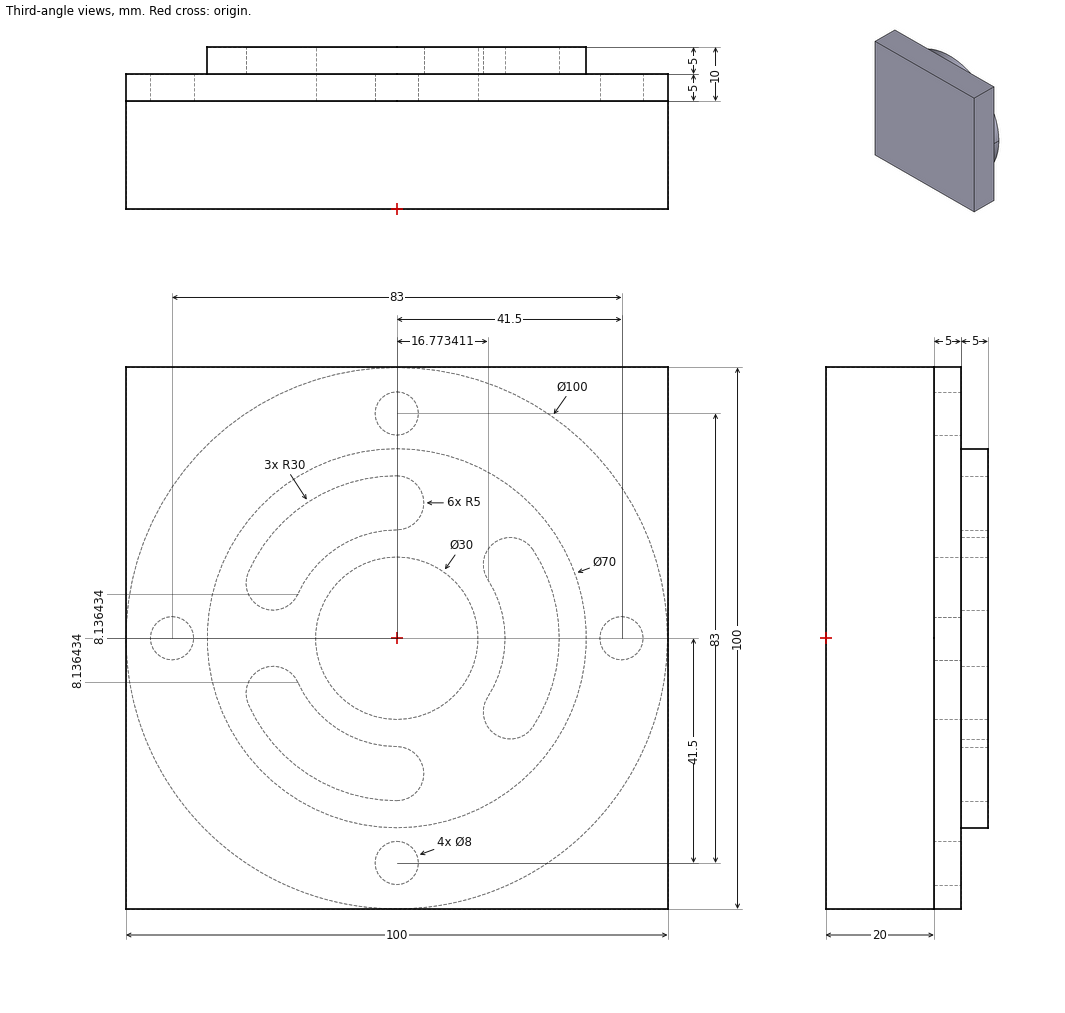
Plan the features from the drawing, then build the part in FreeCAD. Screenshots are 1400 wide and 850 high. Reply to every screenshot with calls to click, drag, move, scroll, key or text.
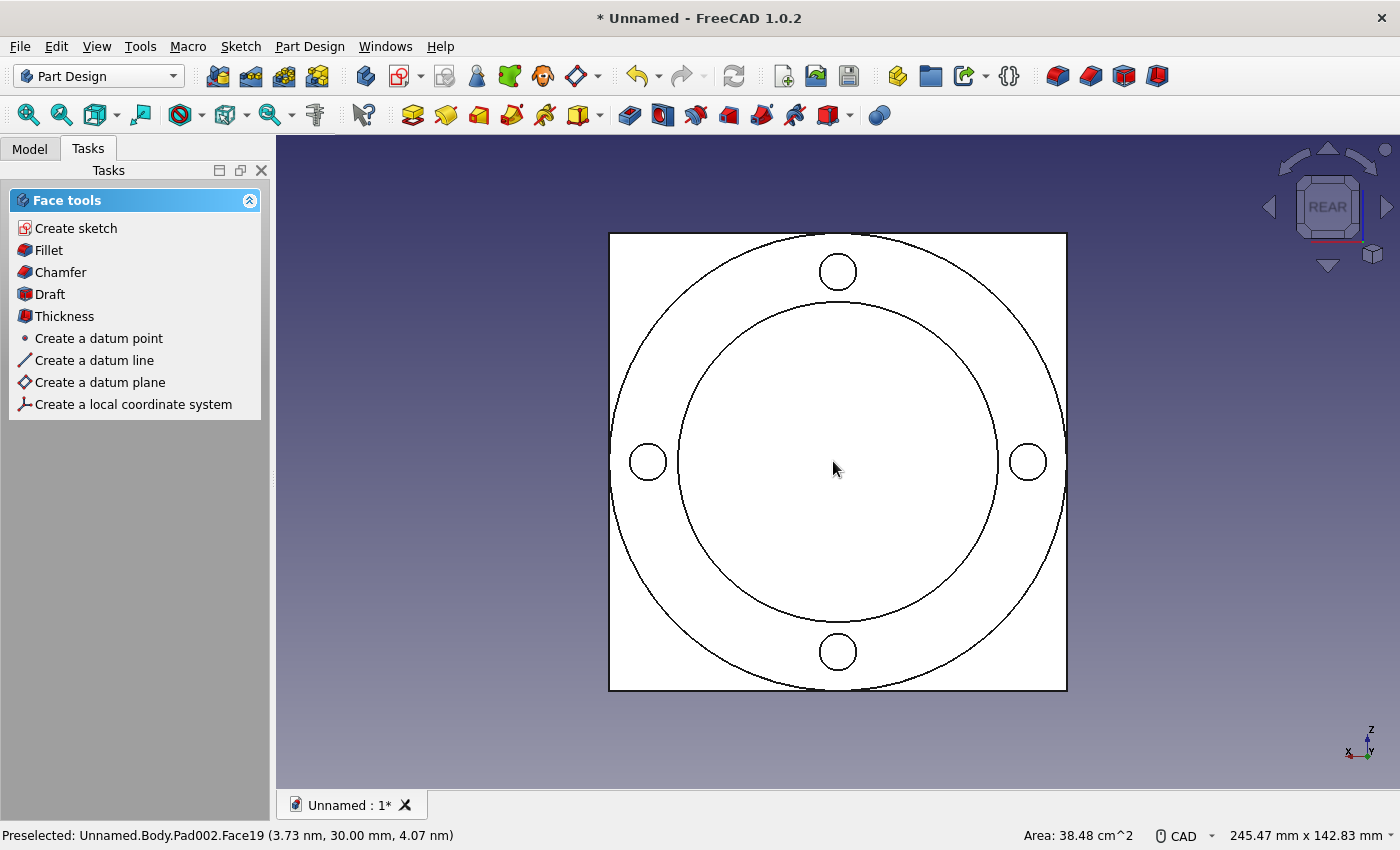
click(398, 76)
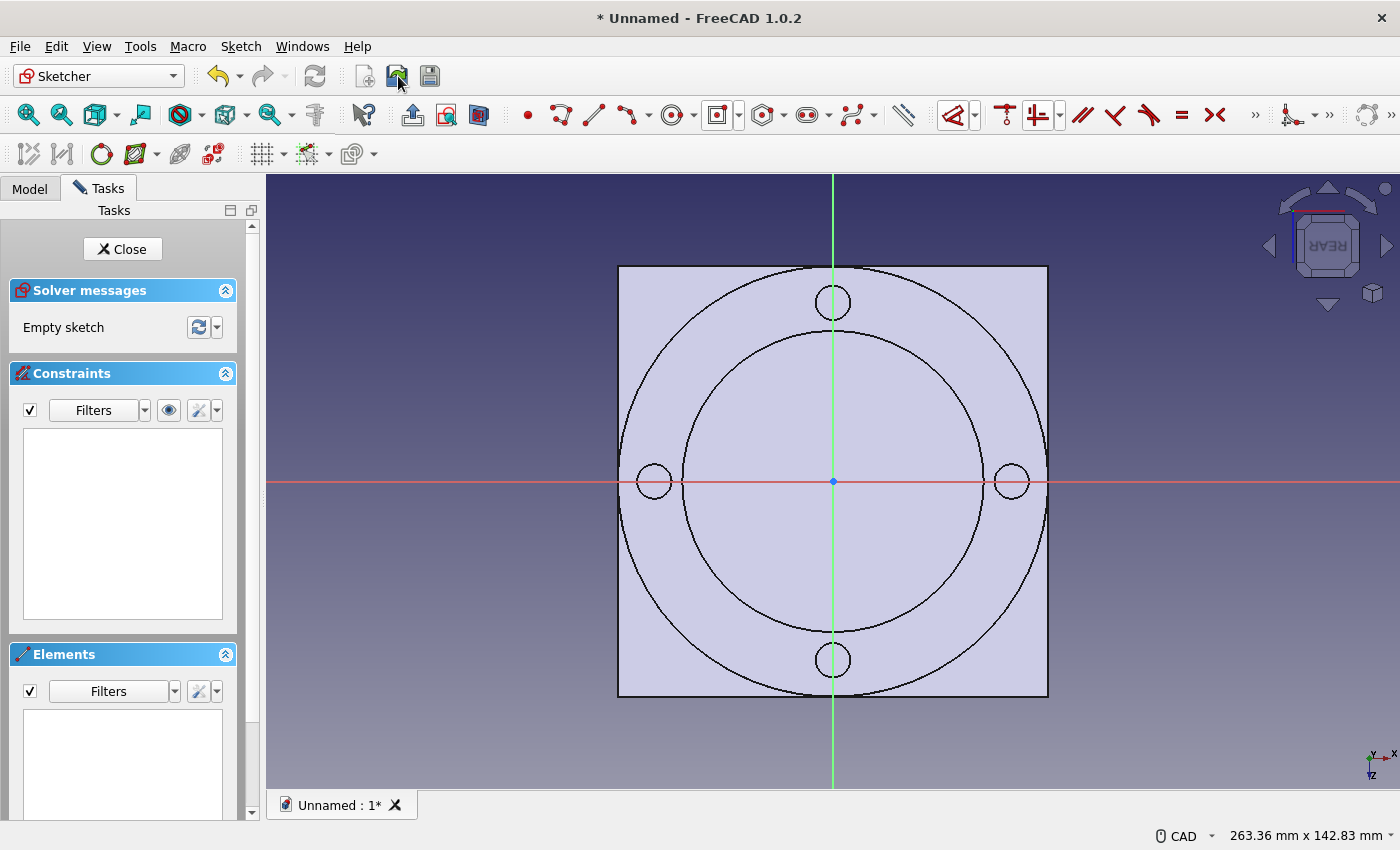
scroll(989, 481, up, 2)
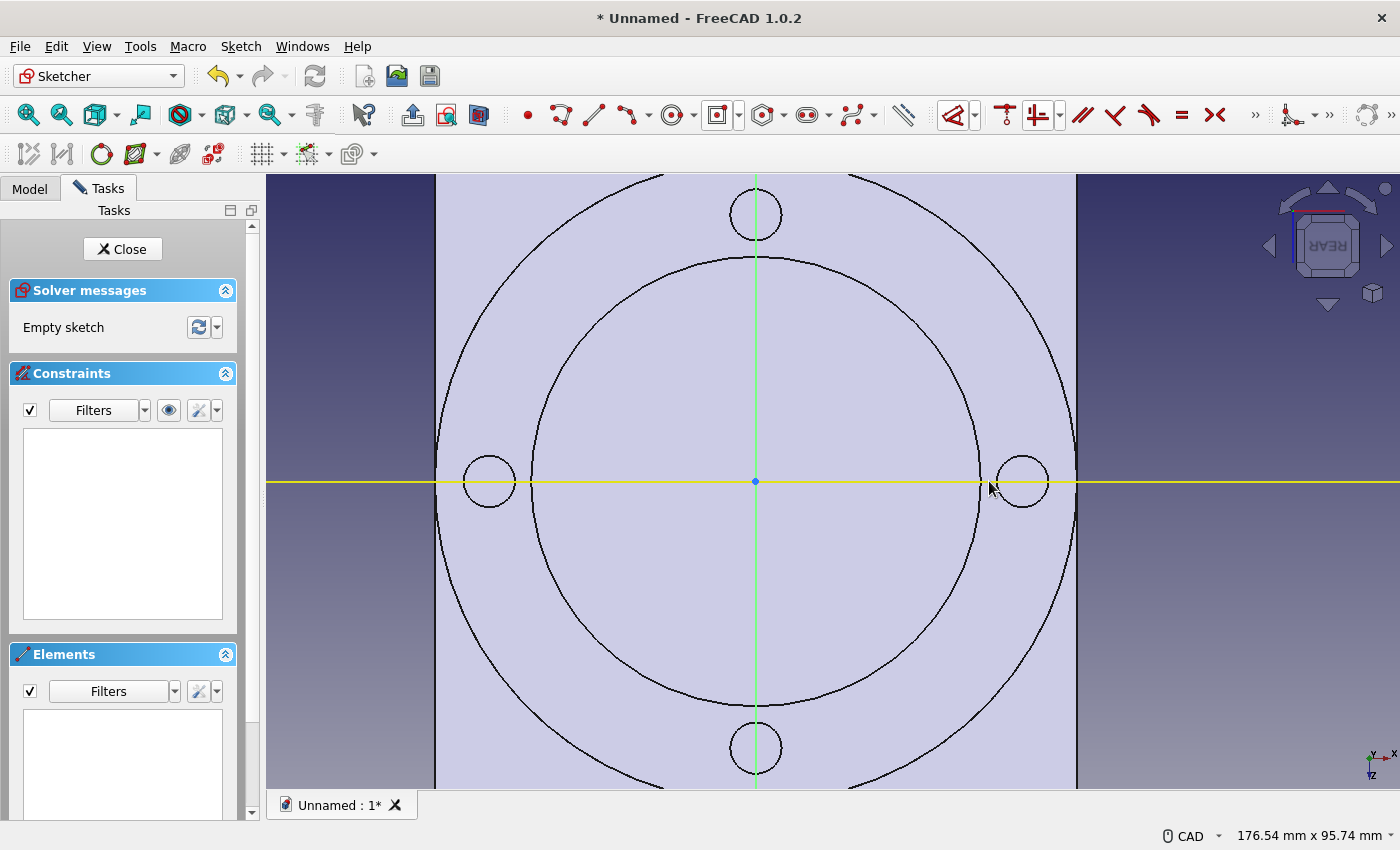
click(626, 116)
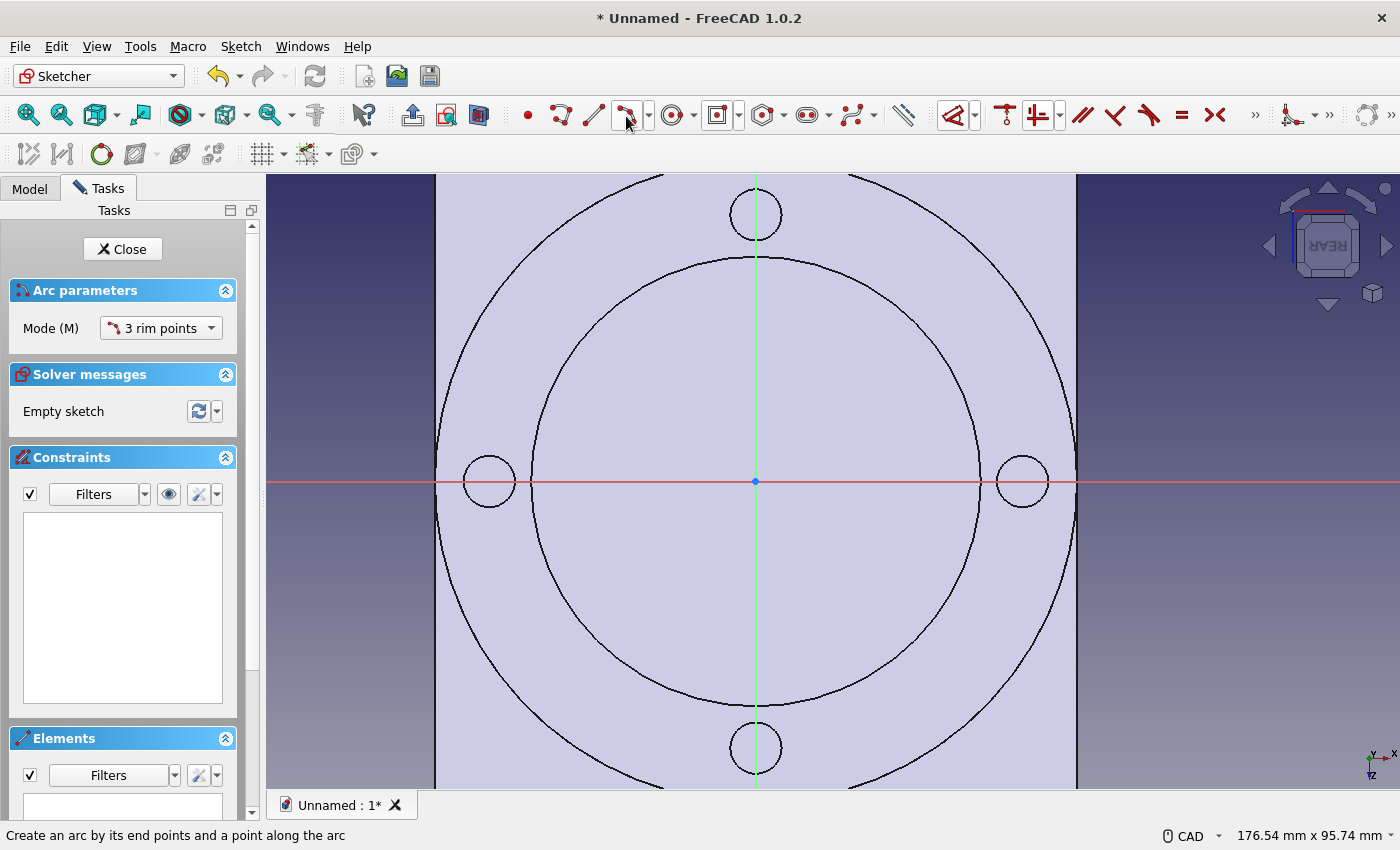
click(639, 534)
click(580, 560)
click(596, 517)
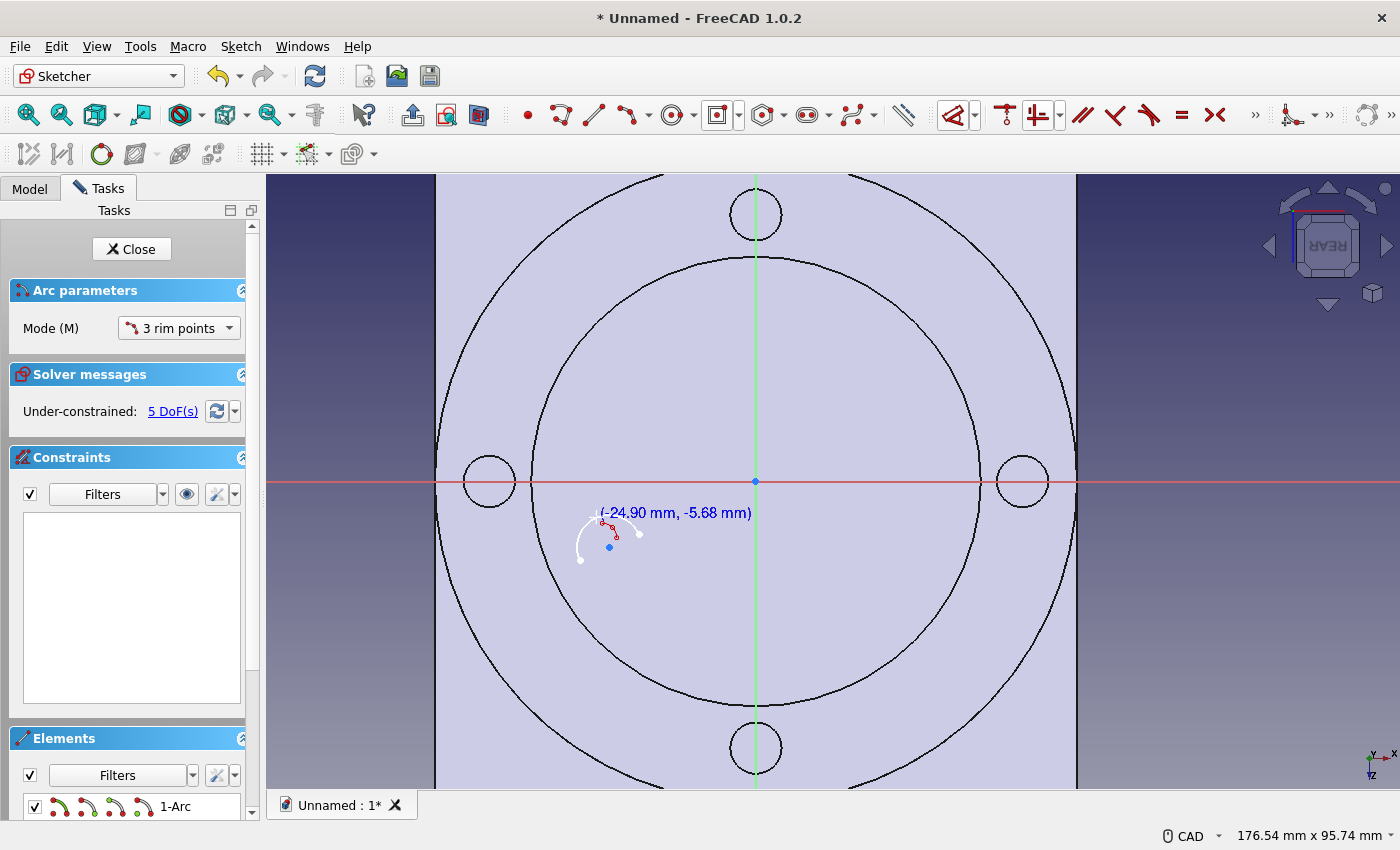
click(580, 561)
click(756, 674)
click(651, 643)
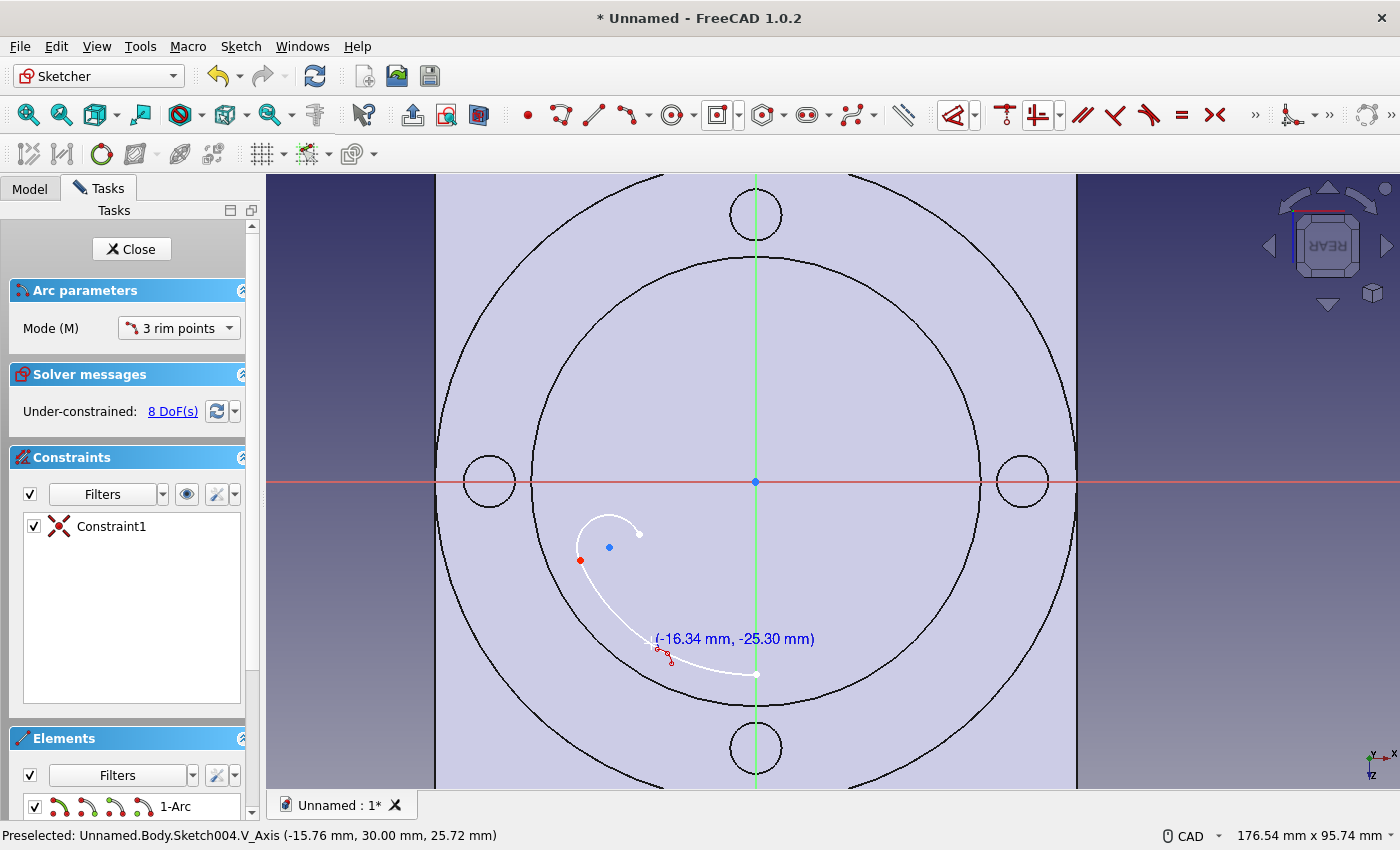
click(756, 675)
click(756, 610)
click(788, 642)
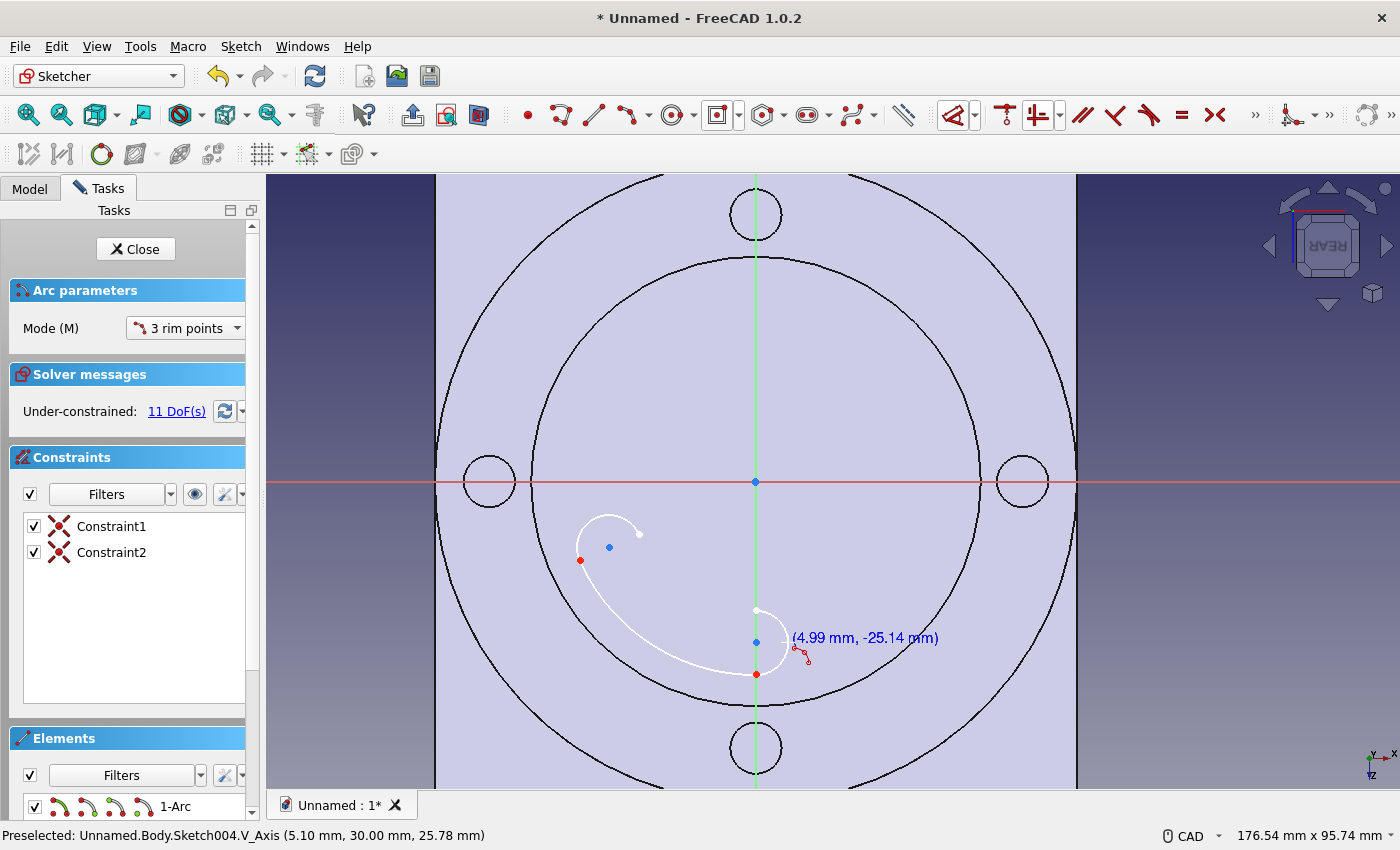
click(756, 611)
click(639, 535)
click(686, 589)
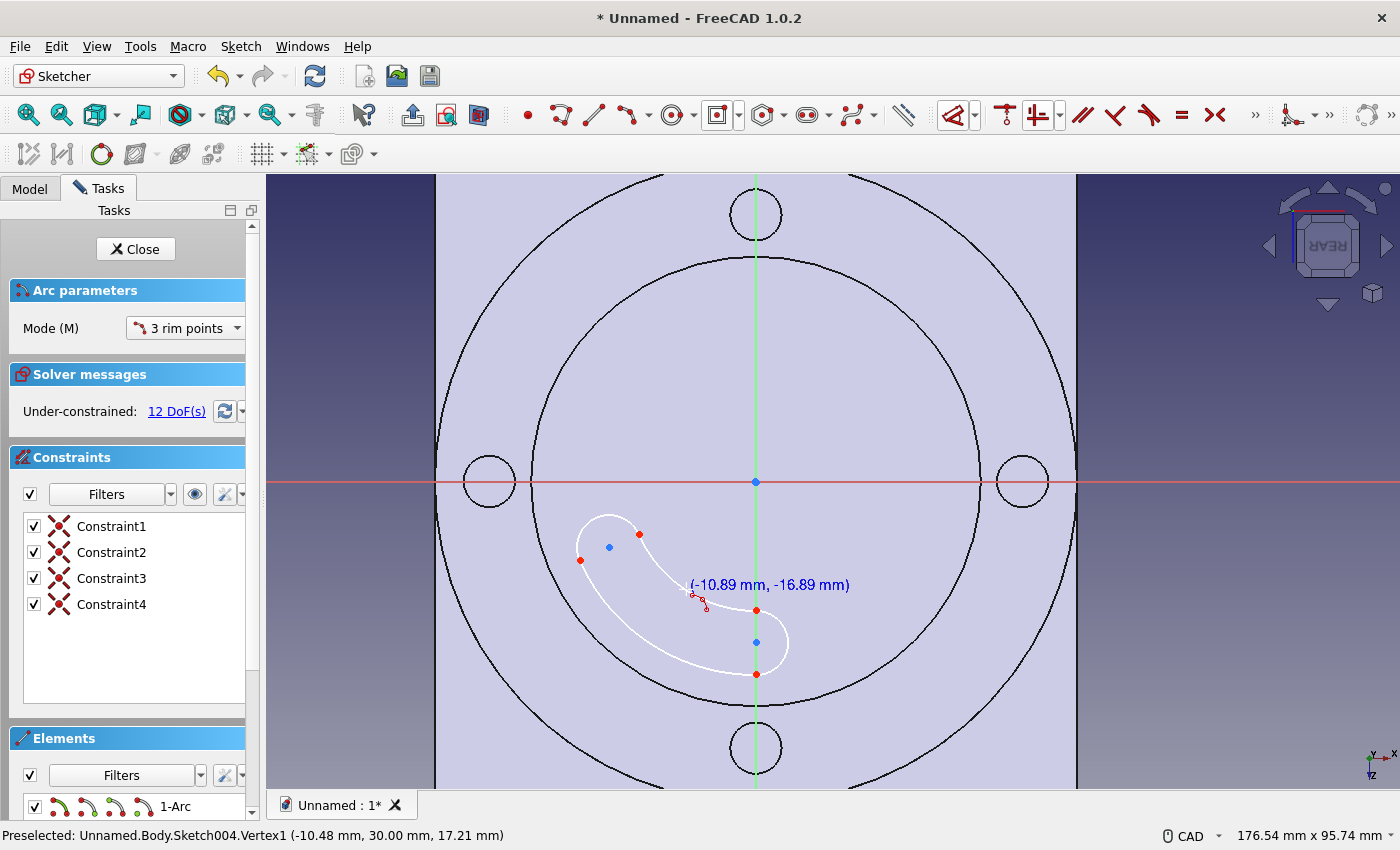
click(864, 412)
click(864, 551)
click(884, 496)